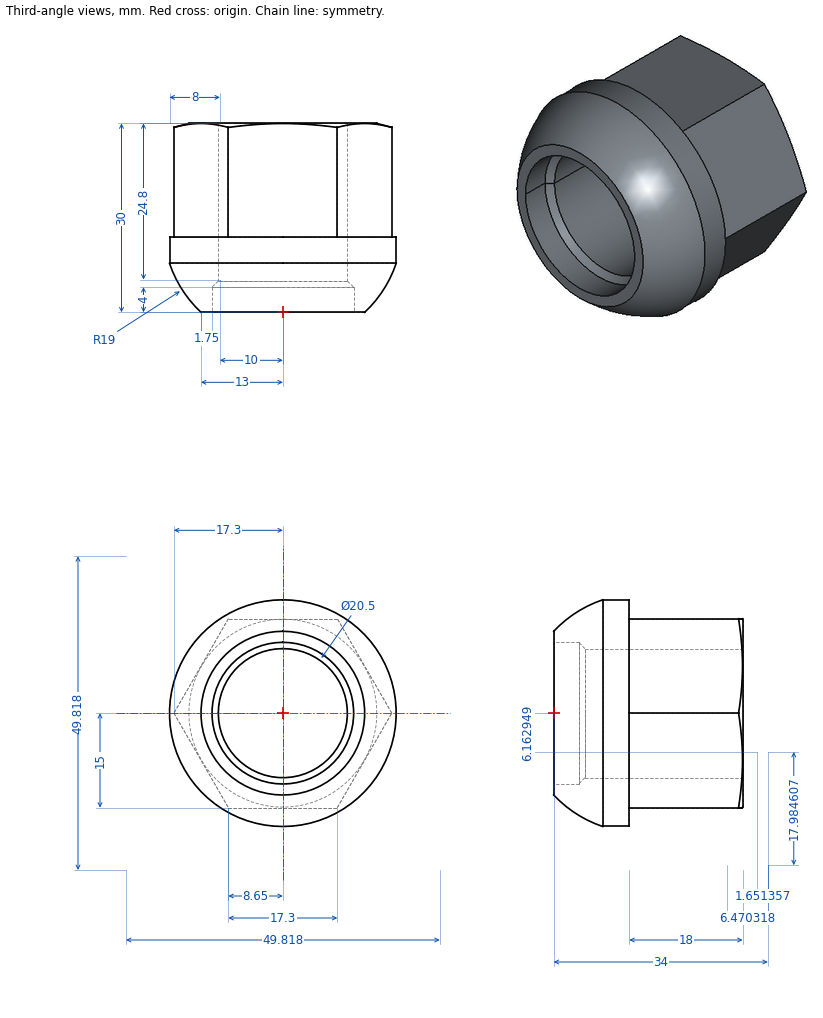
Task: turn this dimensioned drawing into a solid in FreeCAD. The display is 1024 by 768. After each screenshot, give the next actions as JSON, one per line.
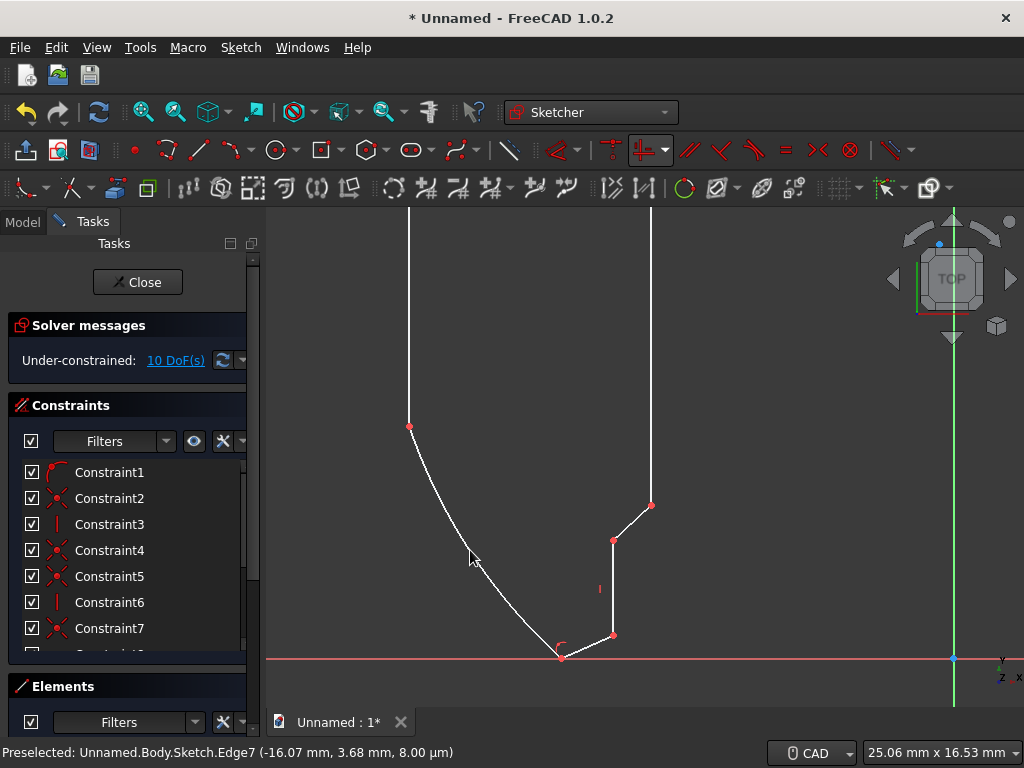
{"action": "left_click", "coordinate": [598, 643]}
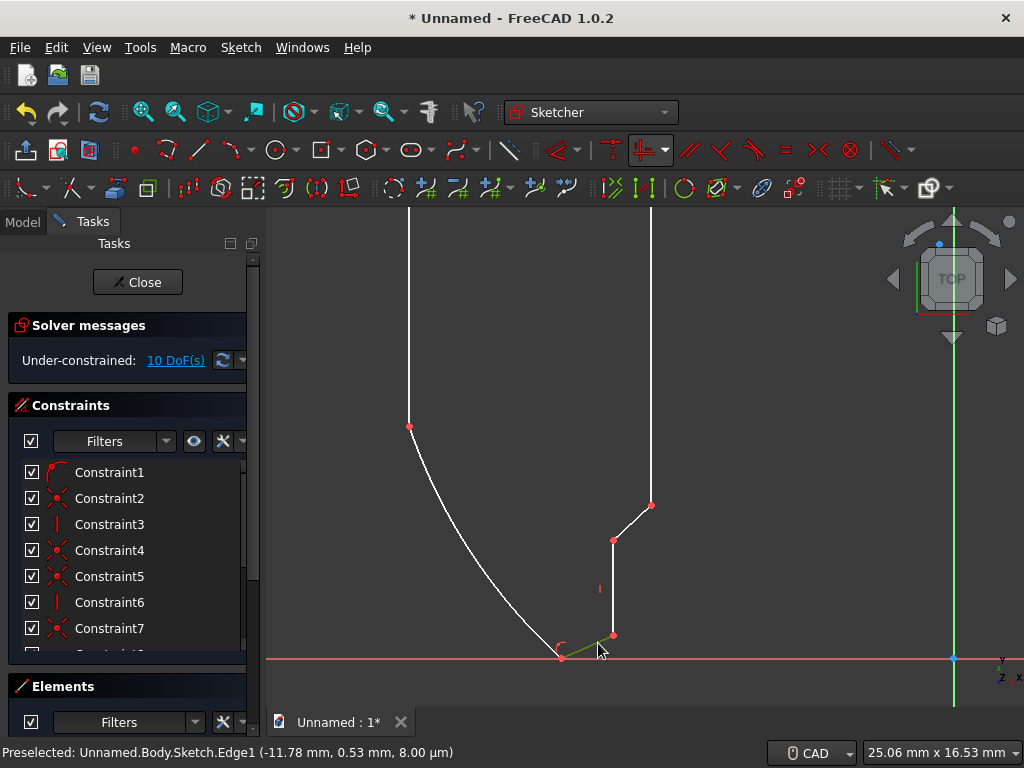
{"action": "key", "text": "h"}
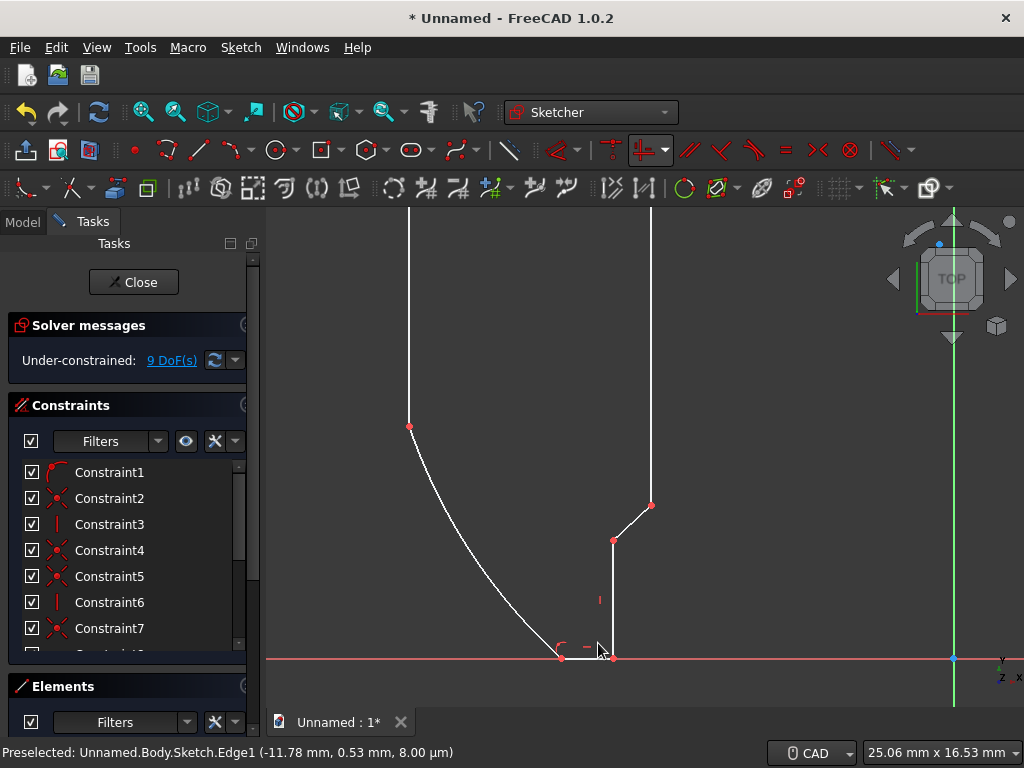
{"action": "scroll", "coordinate": [515, 604], "scroll_direction": "down", "scroll_amount": 5}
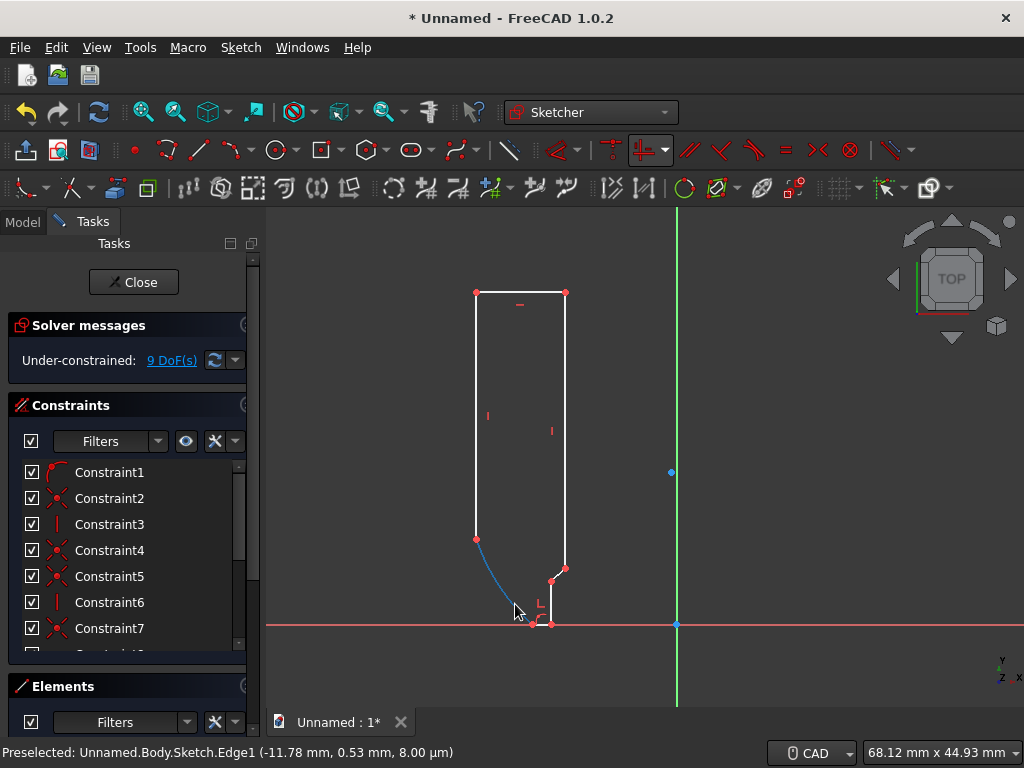
{"action": "left_click", "coordinate": [671, 472]}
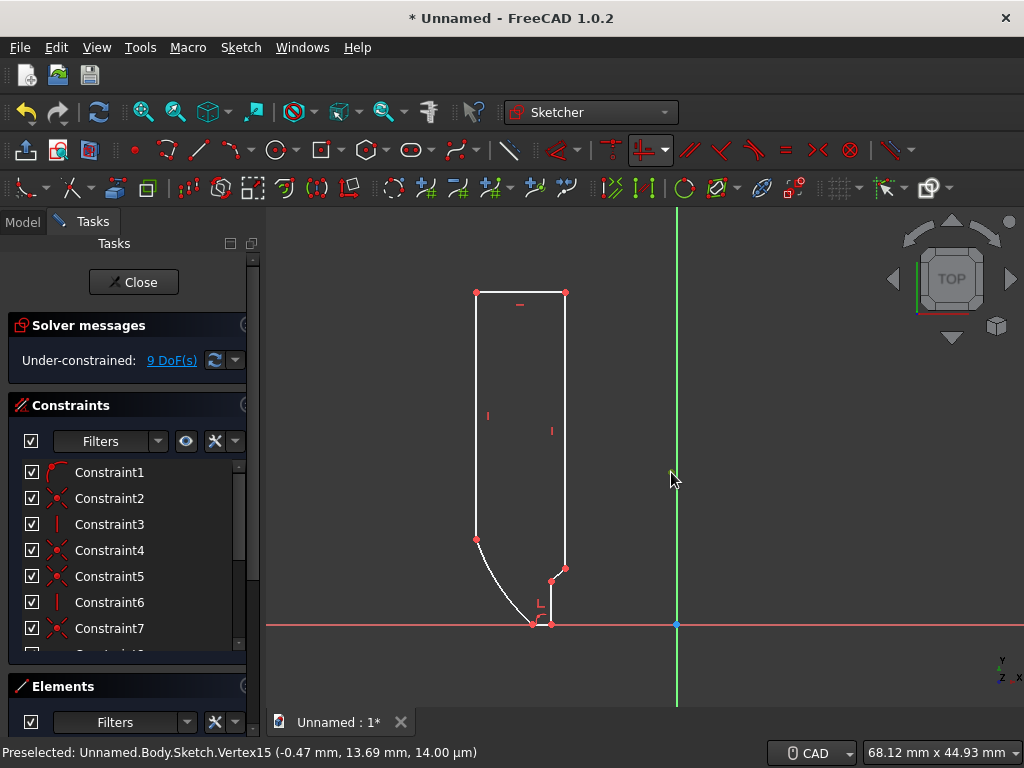
{"action": "left_click", "coordinate": [677, 584]}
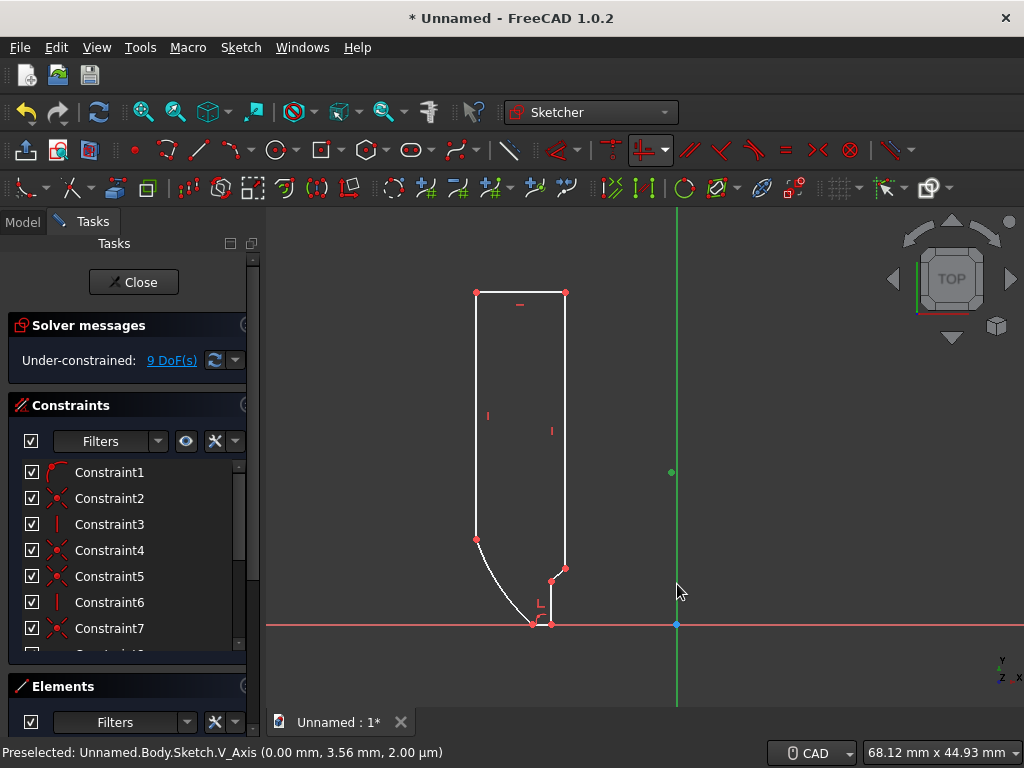
{"action": "key", "text": "c"}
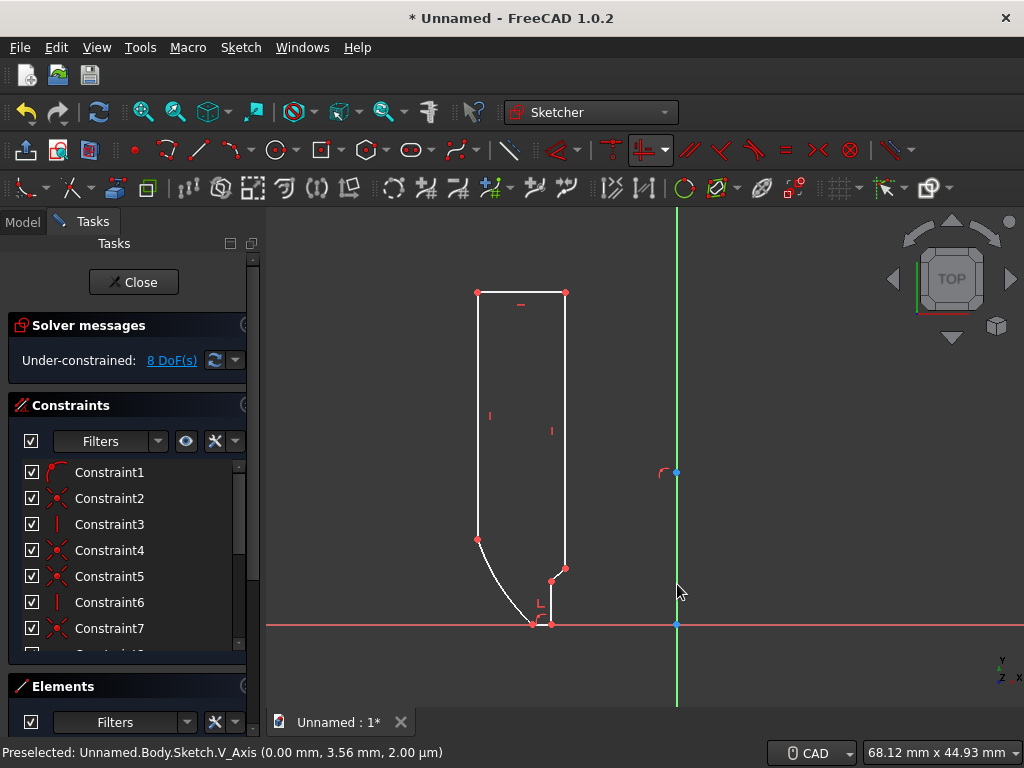
{"action": "left_click", "coordinate": [490, 567]}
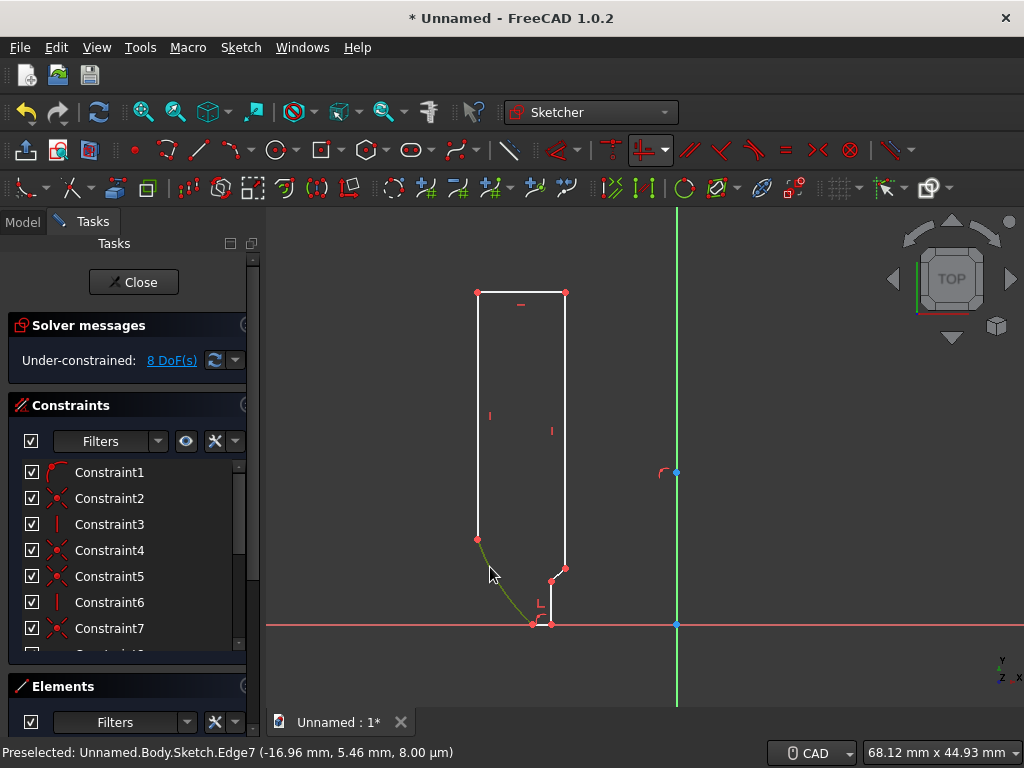
{"action": "key", "text": "k r"}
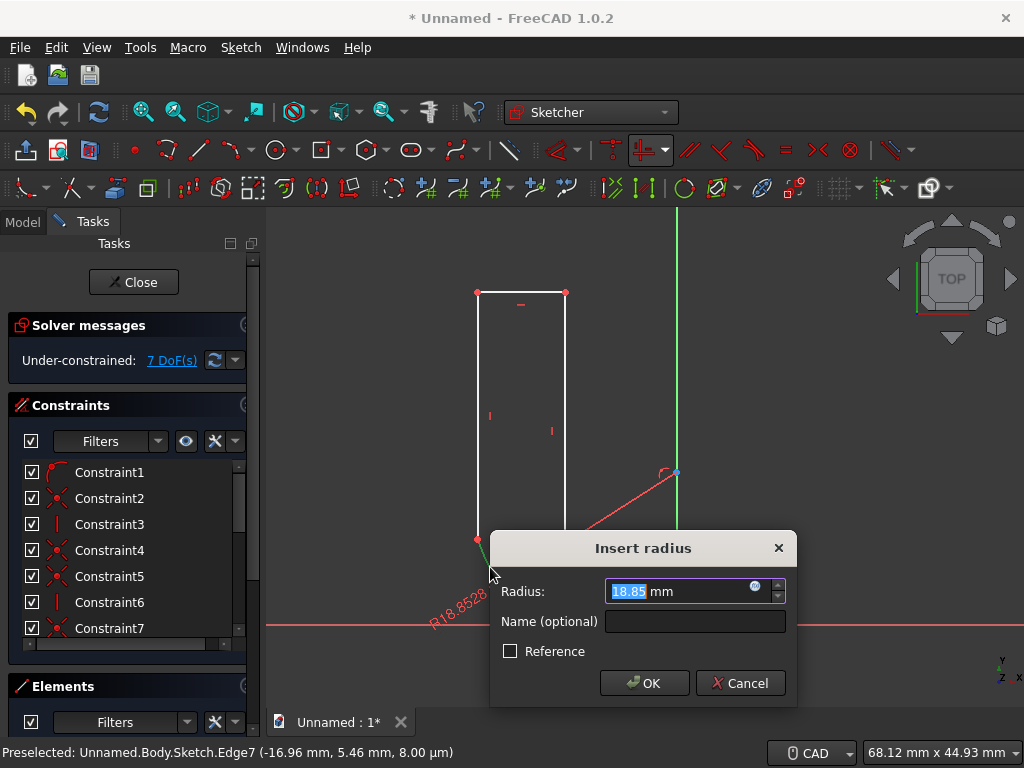
{"action": "type", "text": "19"}
{"action": "key", "text": "Return"}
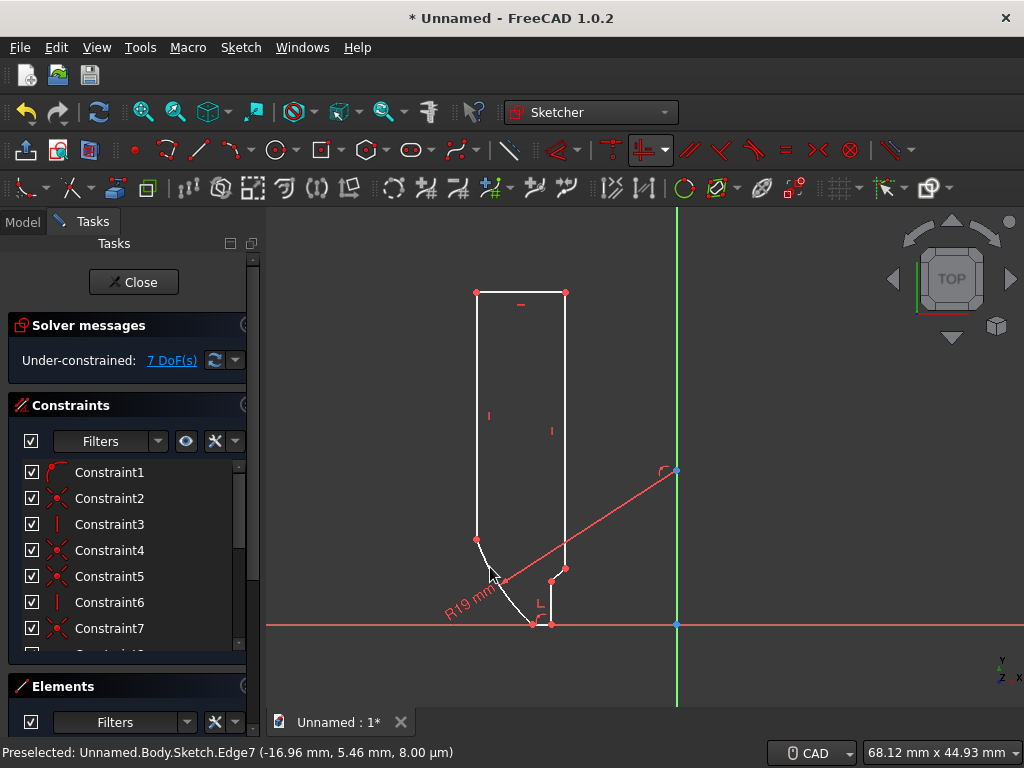
{"action": "left_click", "coordinate": [551, 612]}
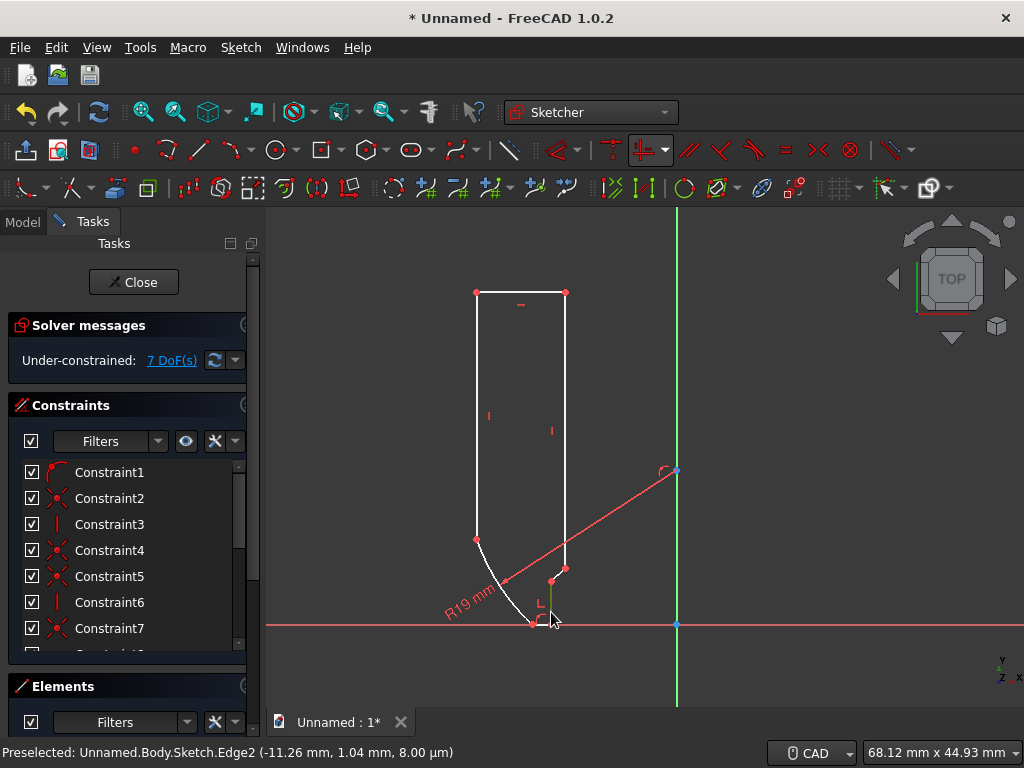
{"action": "key", "text": "i"}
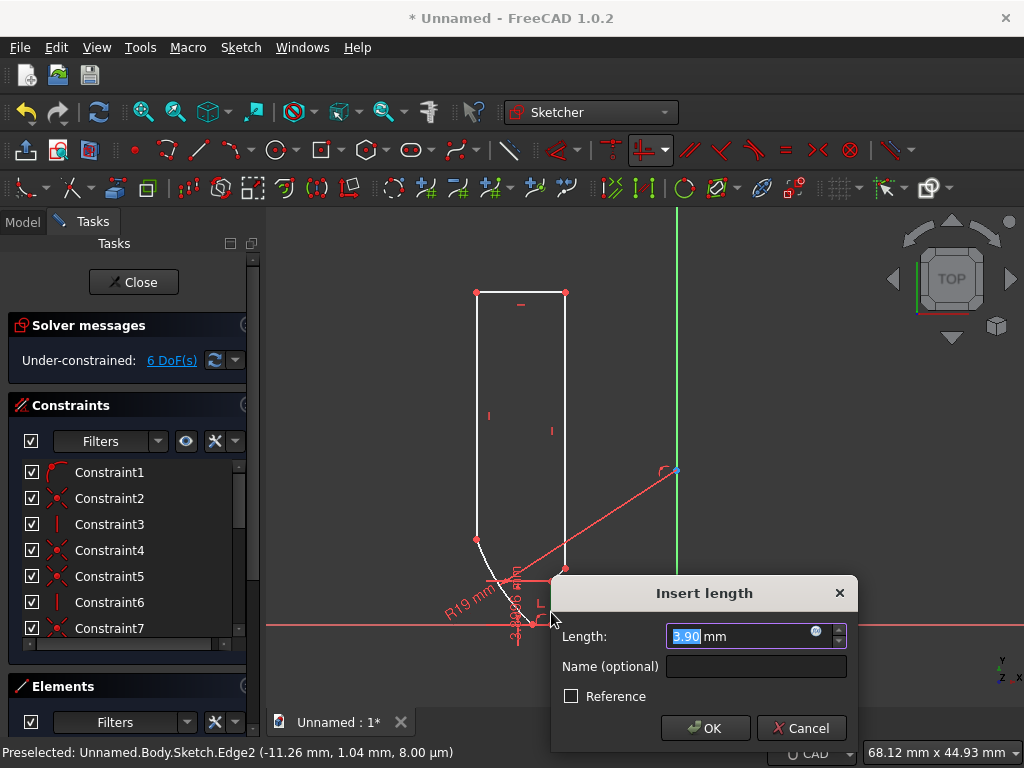
{"action": "type", "text": "4"}
{"action": "key", "text": "Return"}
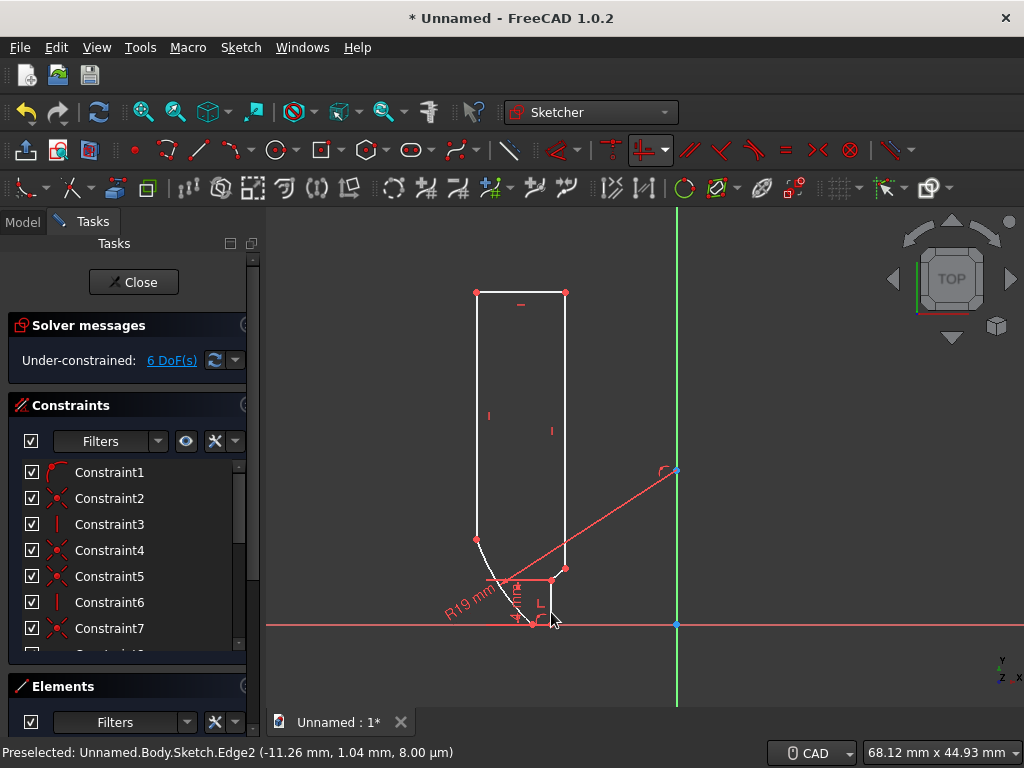
{"action": "left_click", "coordinate": [539, 292]}